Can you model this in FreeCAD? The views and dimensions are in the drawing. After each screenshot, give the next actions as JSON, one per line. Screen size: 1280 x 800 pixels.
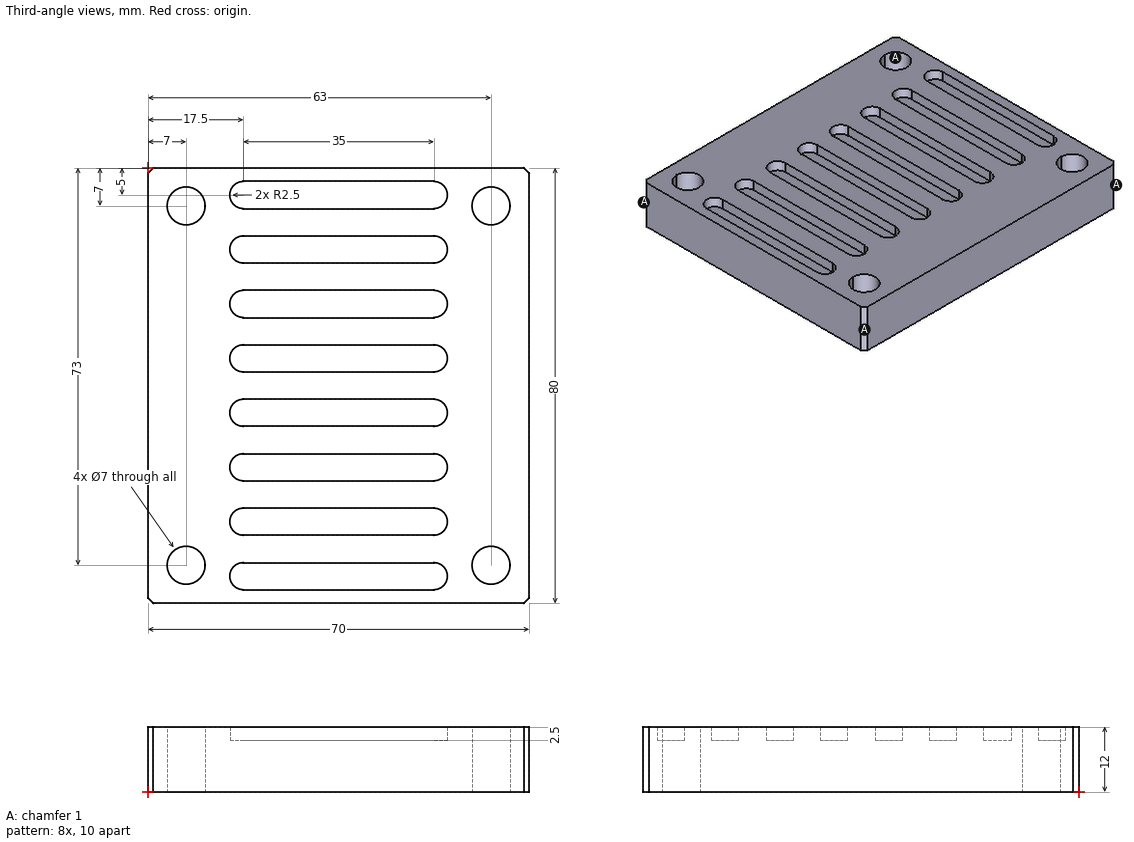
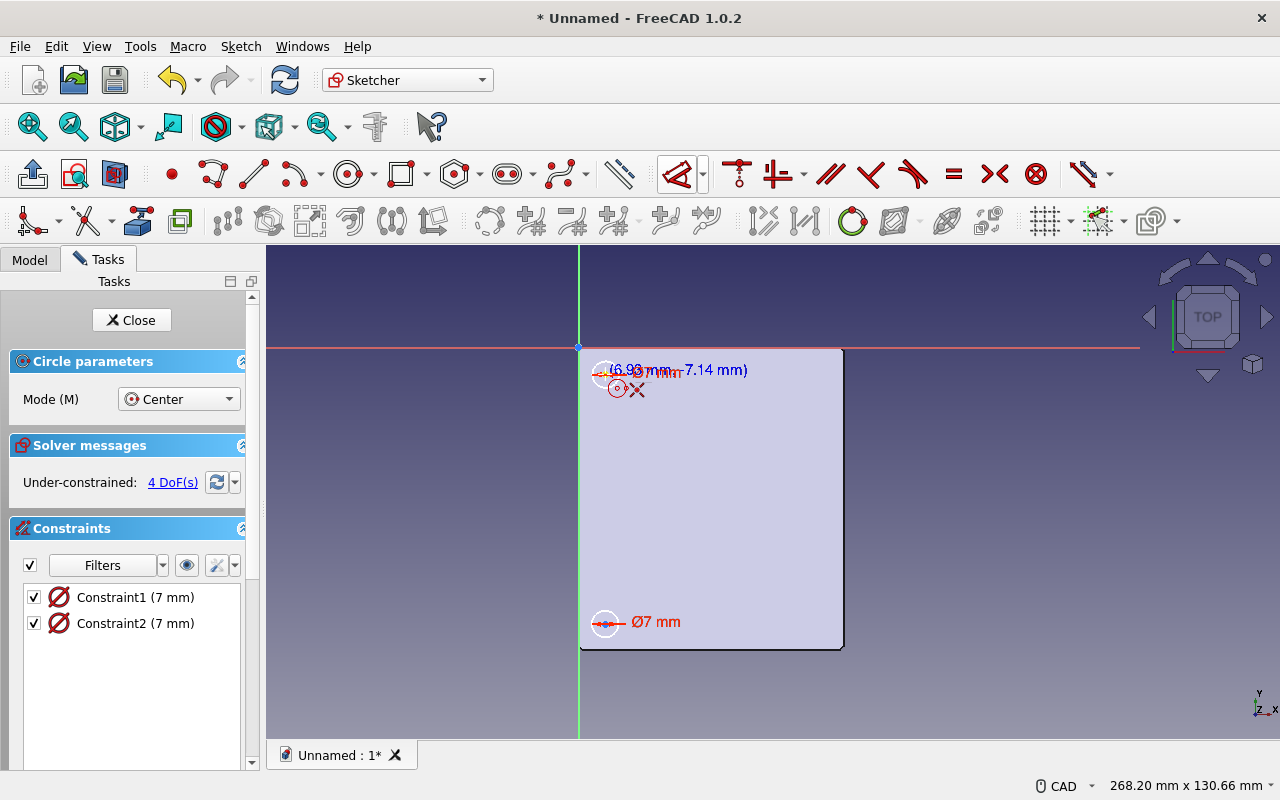
{"action": "scroll", "coordinate": [817, 624], "scroll_direction": "up", "scroll_amount": 3}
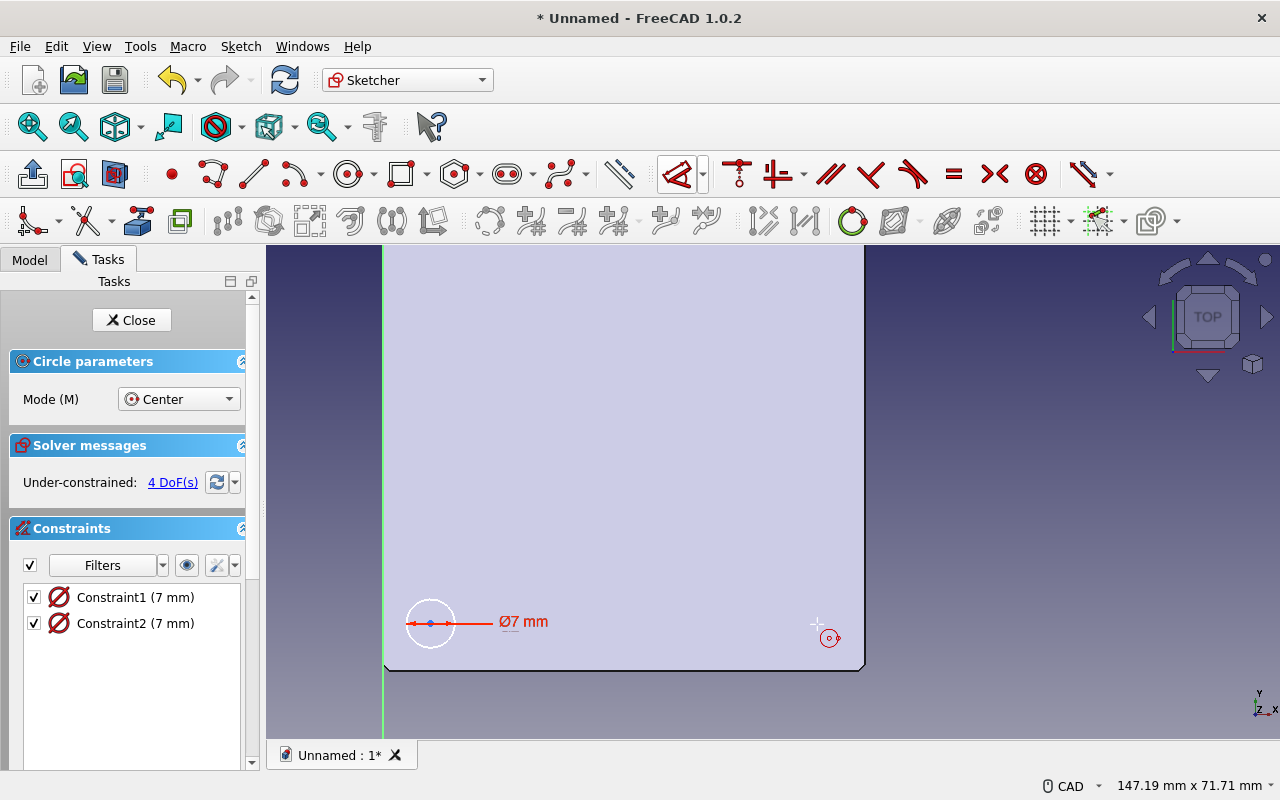
{"action": "left_click", "coordinate": [817, 623]}
{"action": "mouse_move", "coordinate": [834, 606]}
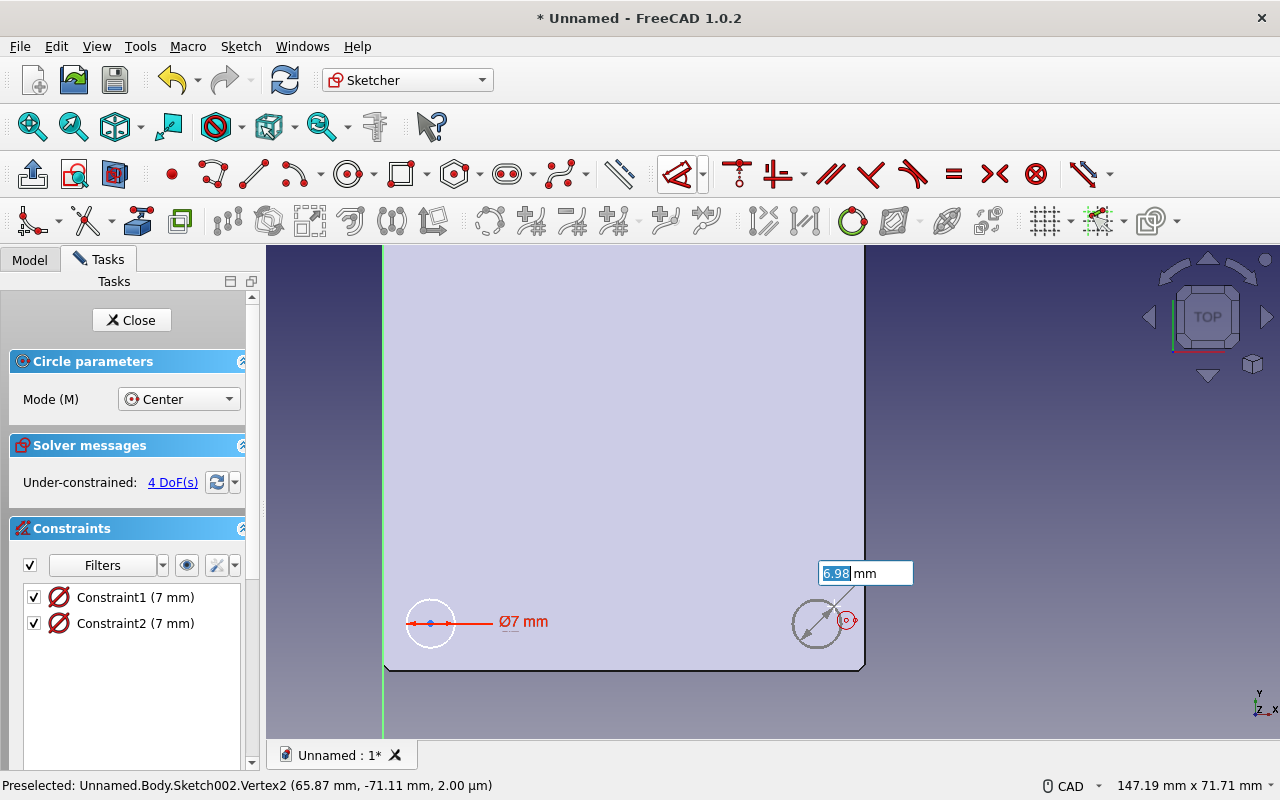
{"action": "type", "text": "7"}
{"action": "key", "text": "Return"}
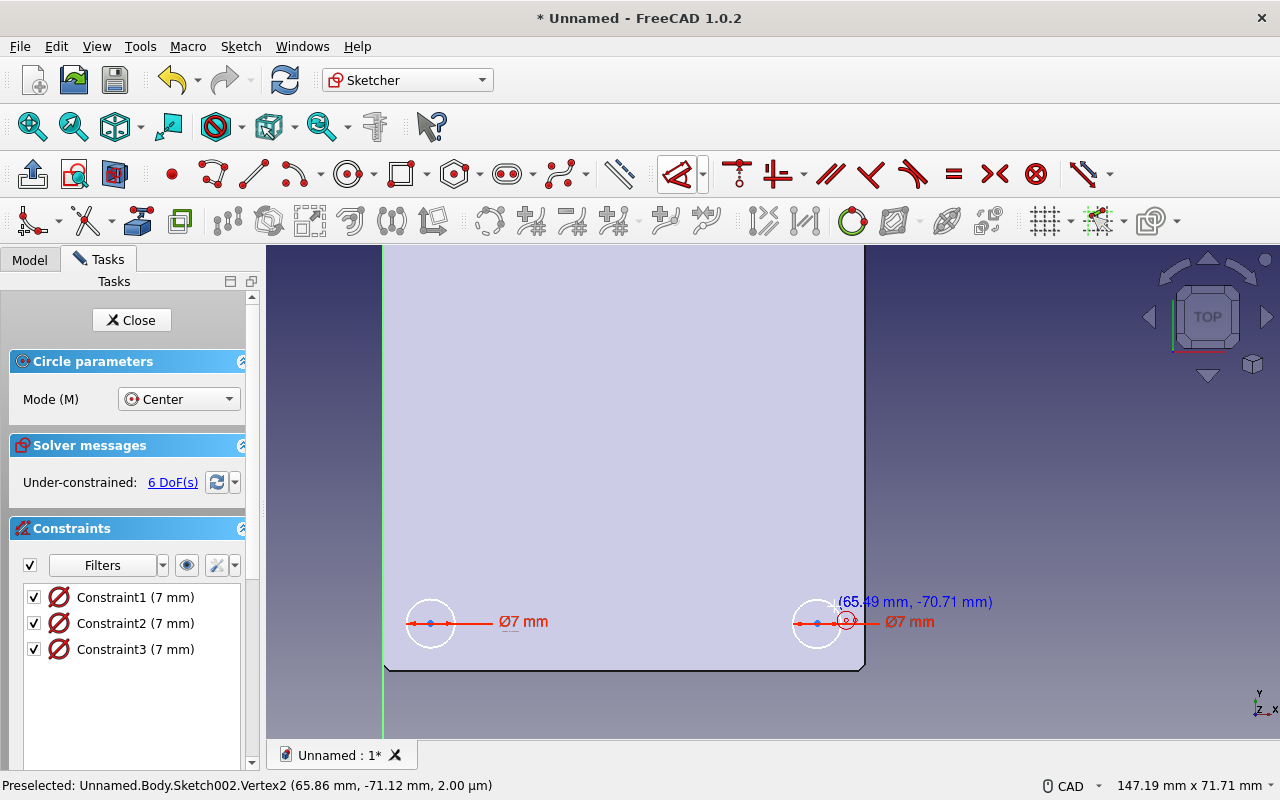
{"action": "scroll", "coordinate": [817, 624], "scroll_direction": "down", "scroll_amount": 3}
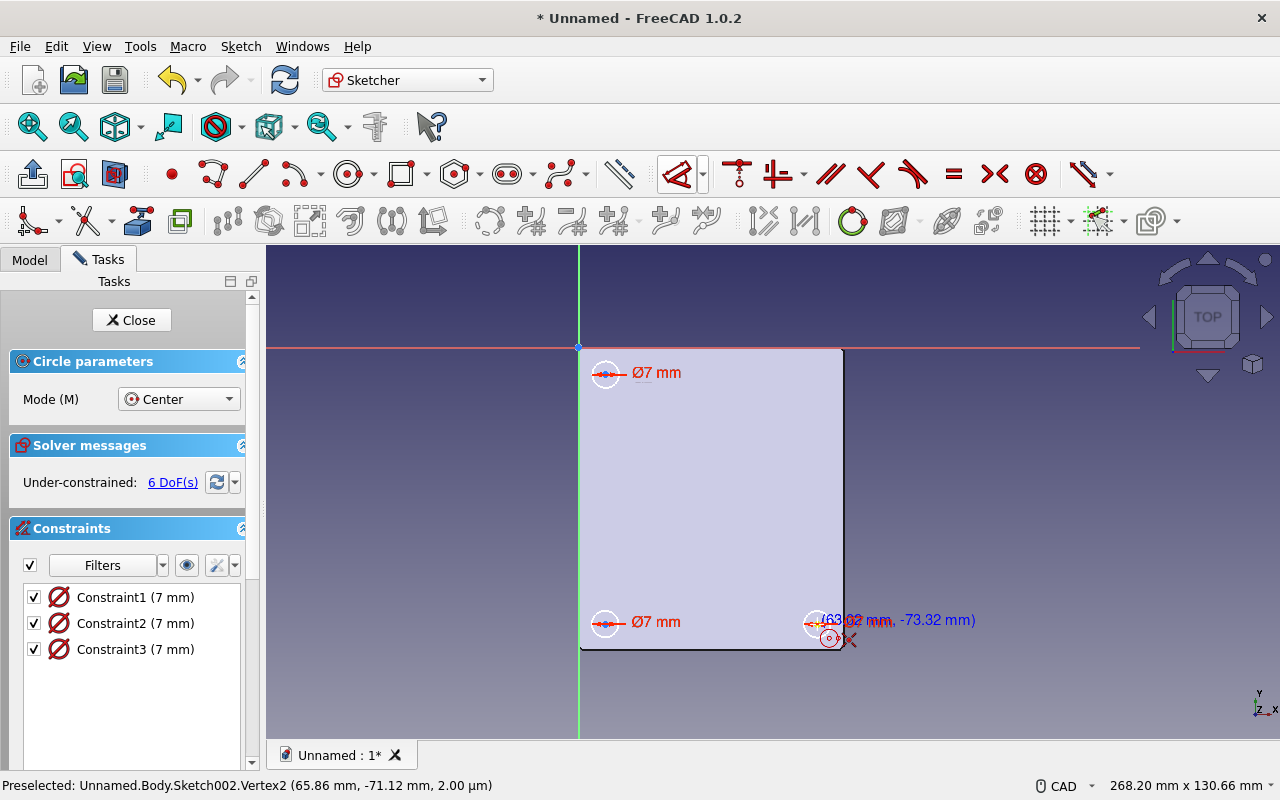
{"action": "scroll", "coordinate": [817, 374], "scroll_direction": "up", "scroll_amount": 3}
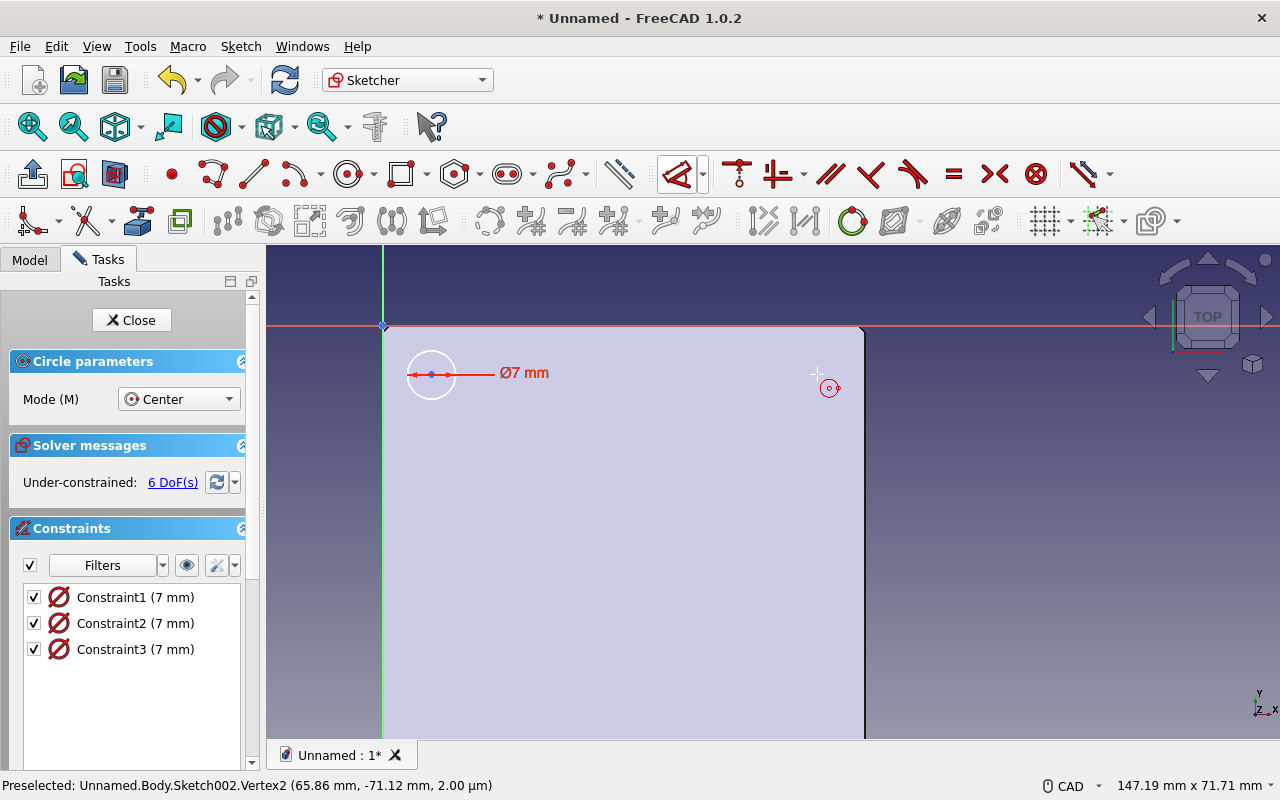
{"action": "left_click", "coordinate": [817, 374]}
{"action": "mouse_move", "coordinate": [834, 357]}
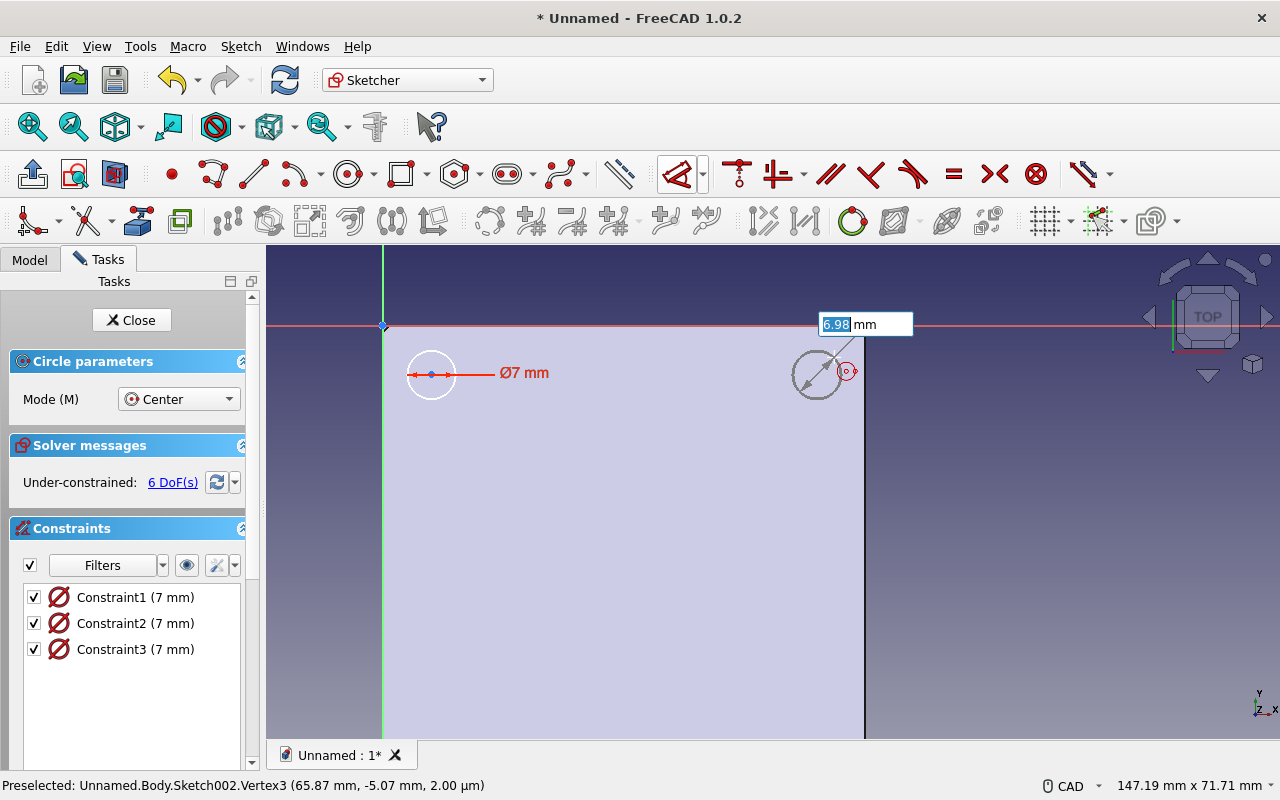
{"action": "type", "text": "7"}
{"action": "key", "text": "Return"}
{"action": "key", "text": "Escape"}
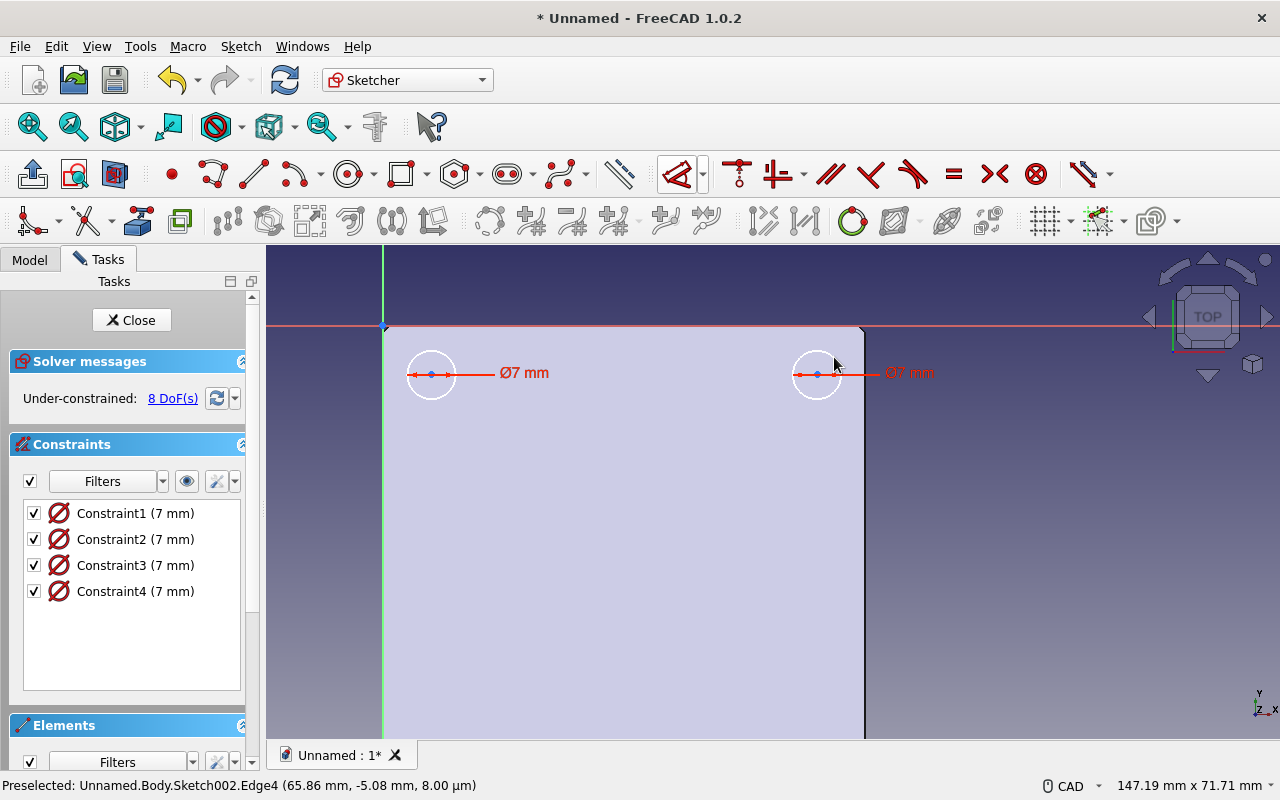
{"action": "key", "text": "d"}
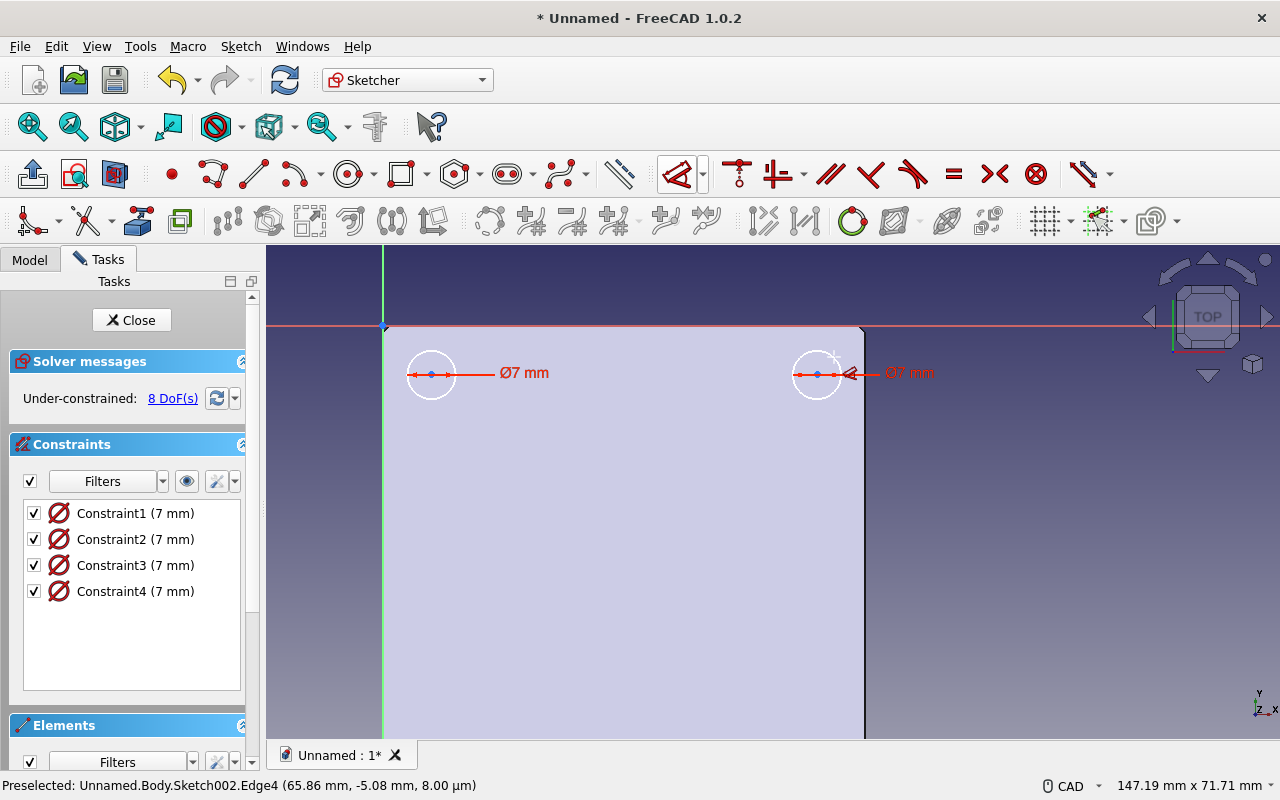
{"action": "scroll", "coordinate": [817, 374], "scroll_direction": "down", "scroll_amount": 3}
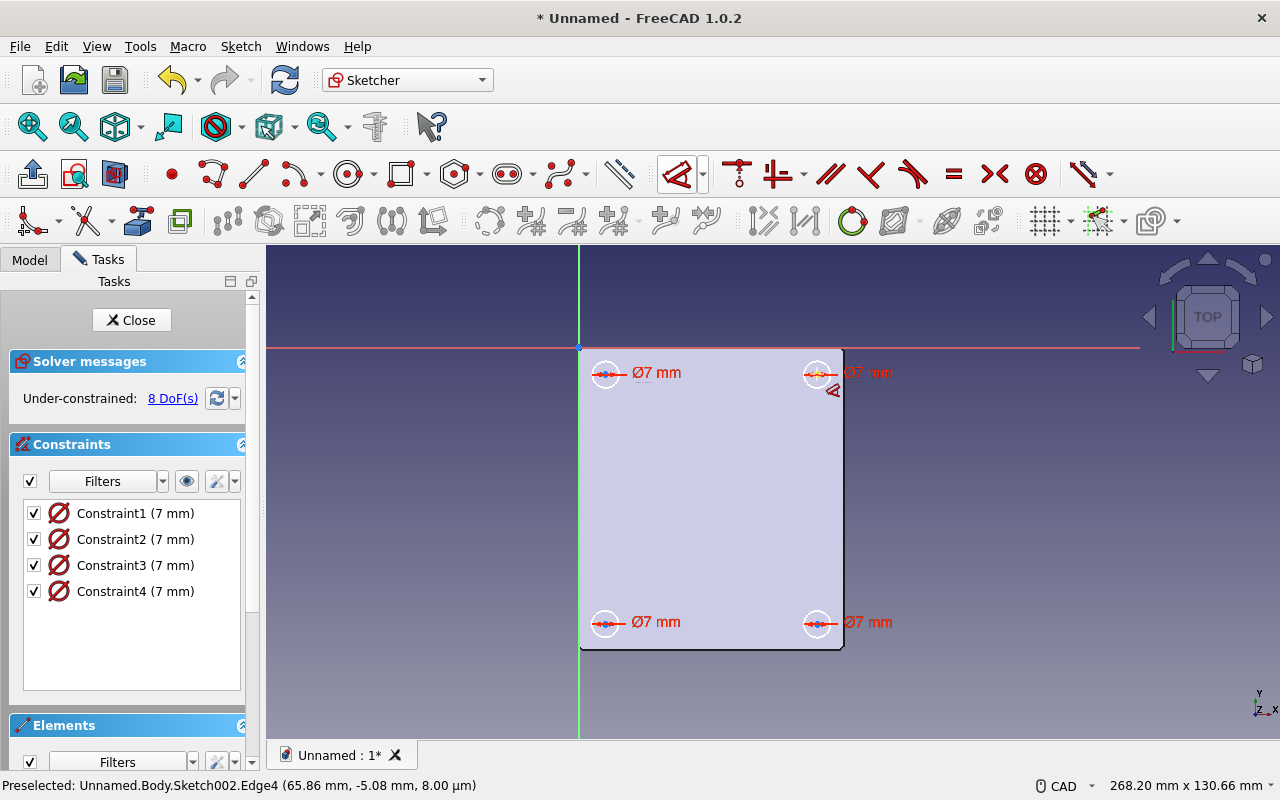
{"action": "scroll", "coordinate": [605, 624], "scroll_direction": "up", "scroll_amount": 3}